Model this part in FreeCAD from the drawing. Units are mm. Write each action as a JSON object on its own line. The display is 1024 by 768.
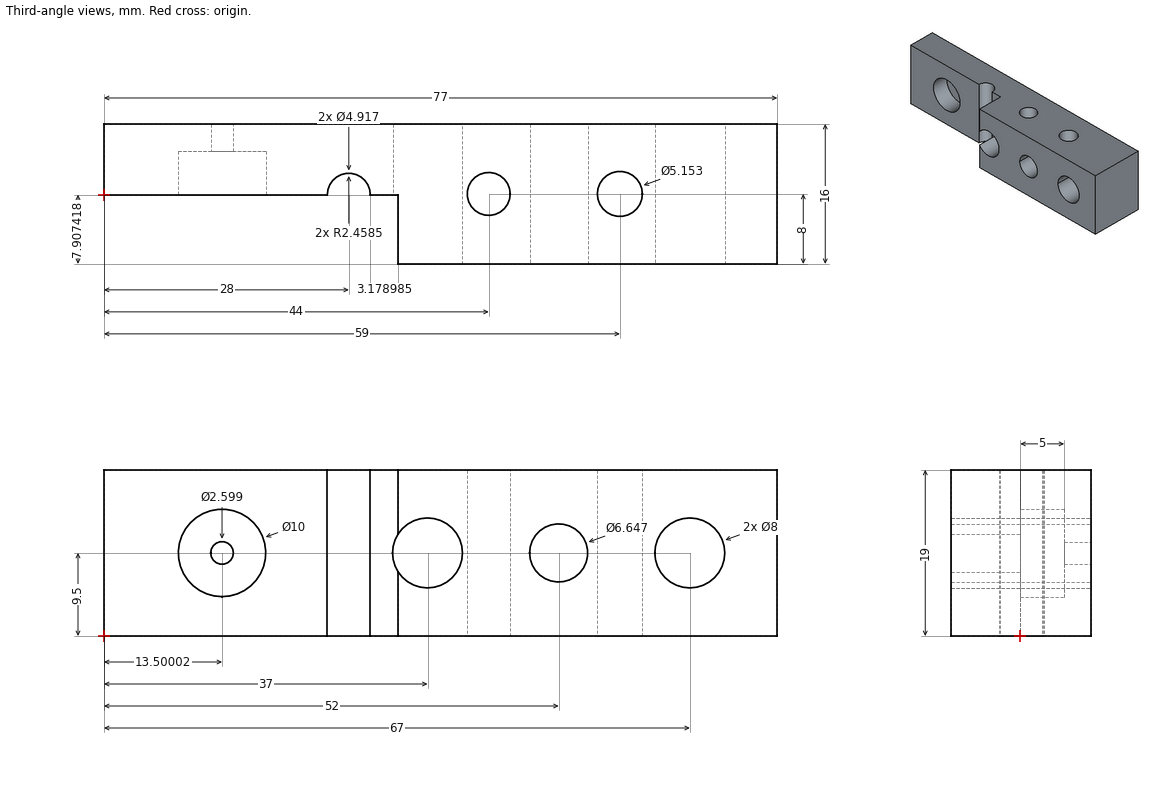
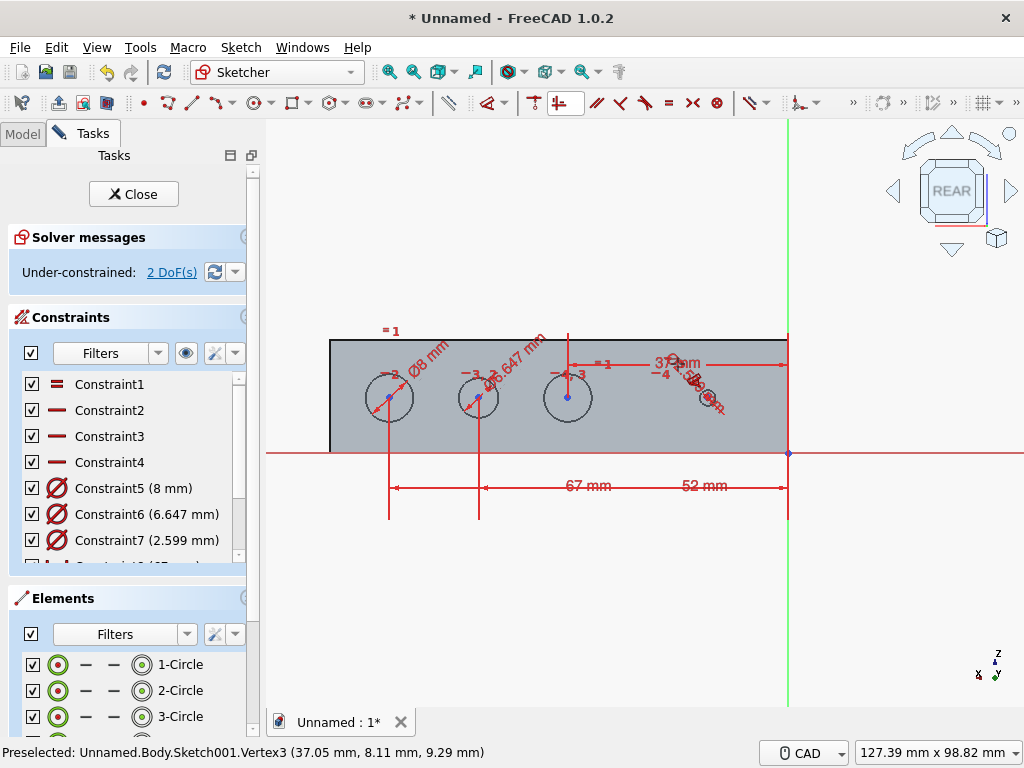
{"action": "left_click", "coordinate": [389, 398]}
{"action": "left_click", "coordinate": [822, 426]}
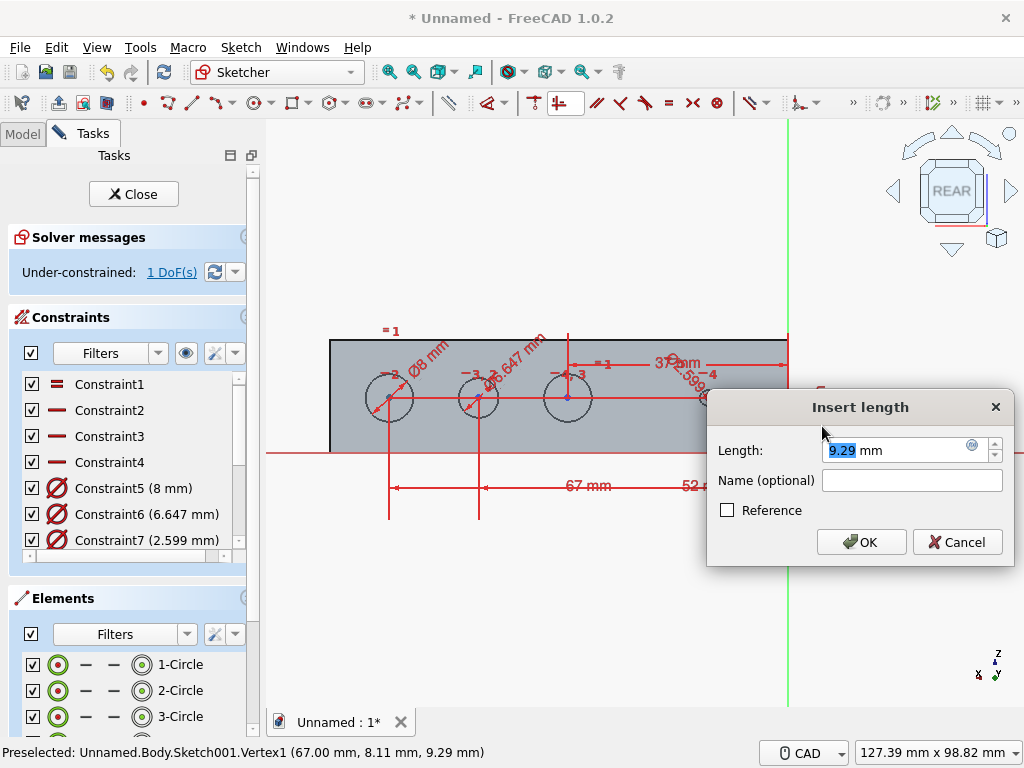
{"action": "type", "text": "9.5"}
{"action": "key", "text": "Return"}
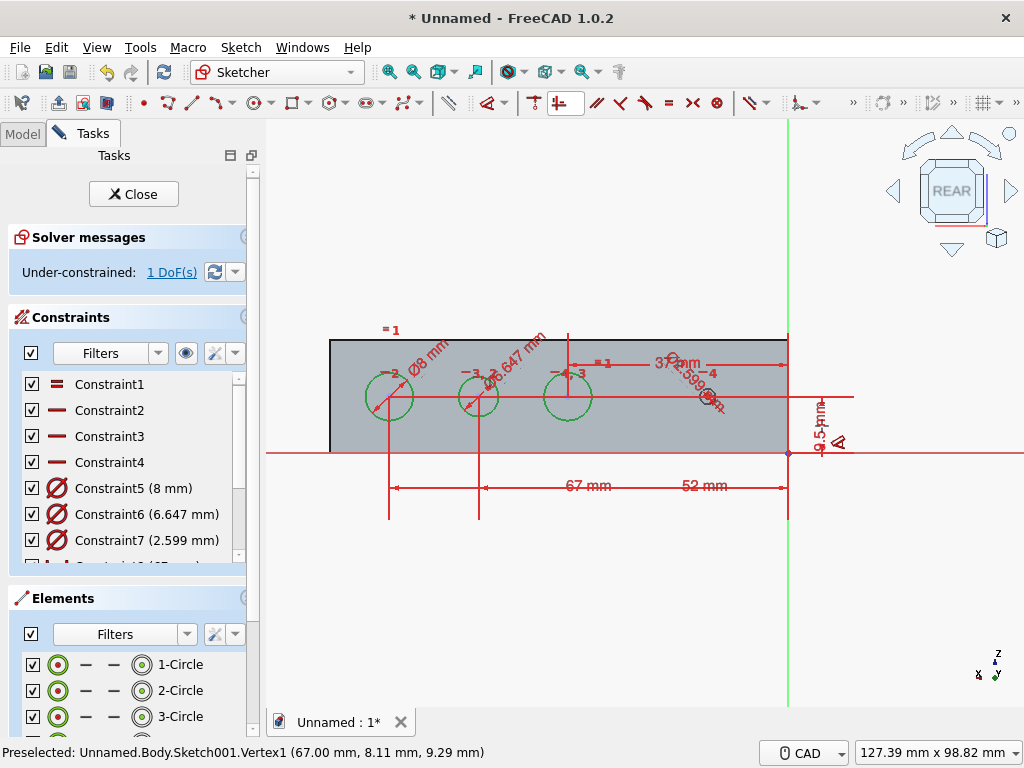
{"action": "left_click", "coordinate": [708, 397]}
{"action": "left_click", "coordinate": [748, 363]}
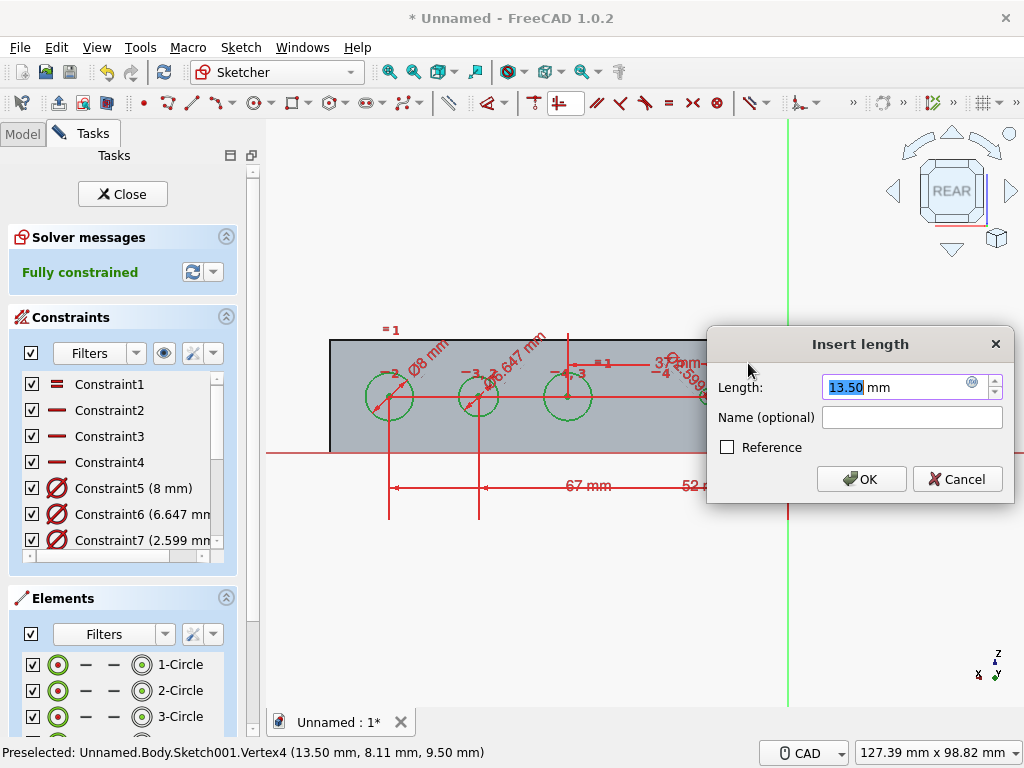
{"action": "type", "text": "13.50002"}
{"action": "key", "text": "Return"}
{"action": "key", "text": "Escape"}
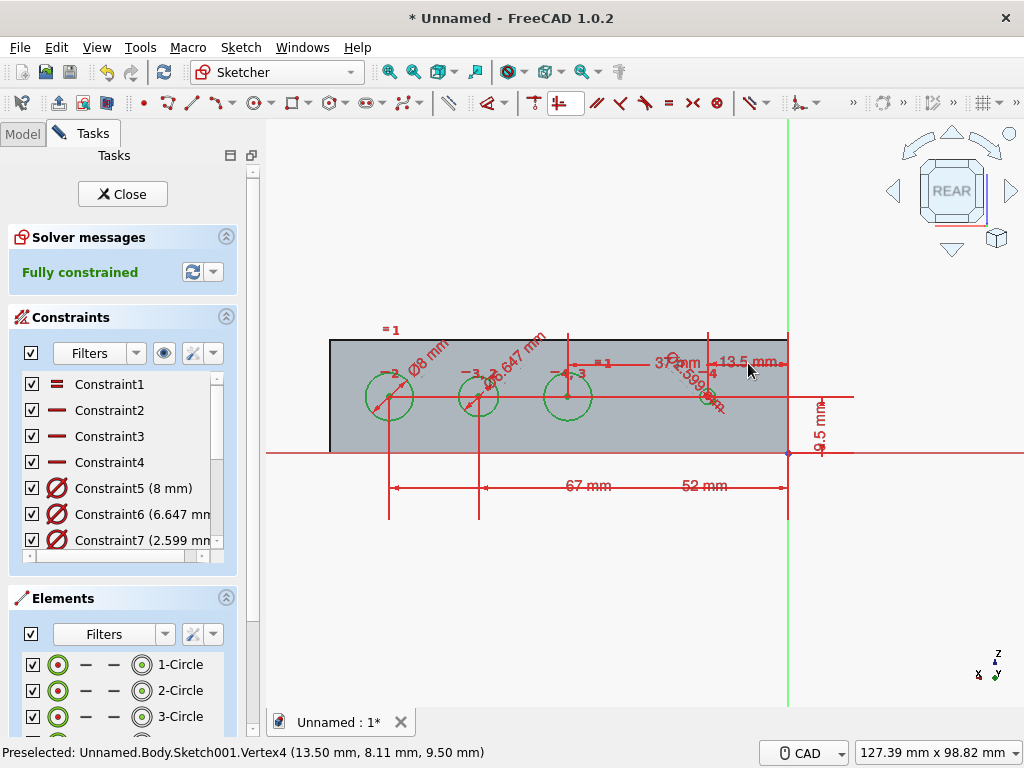
{"action": "left_click", "coordinate": [123, 194]}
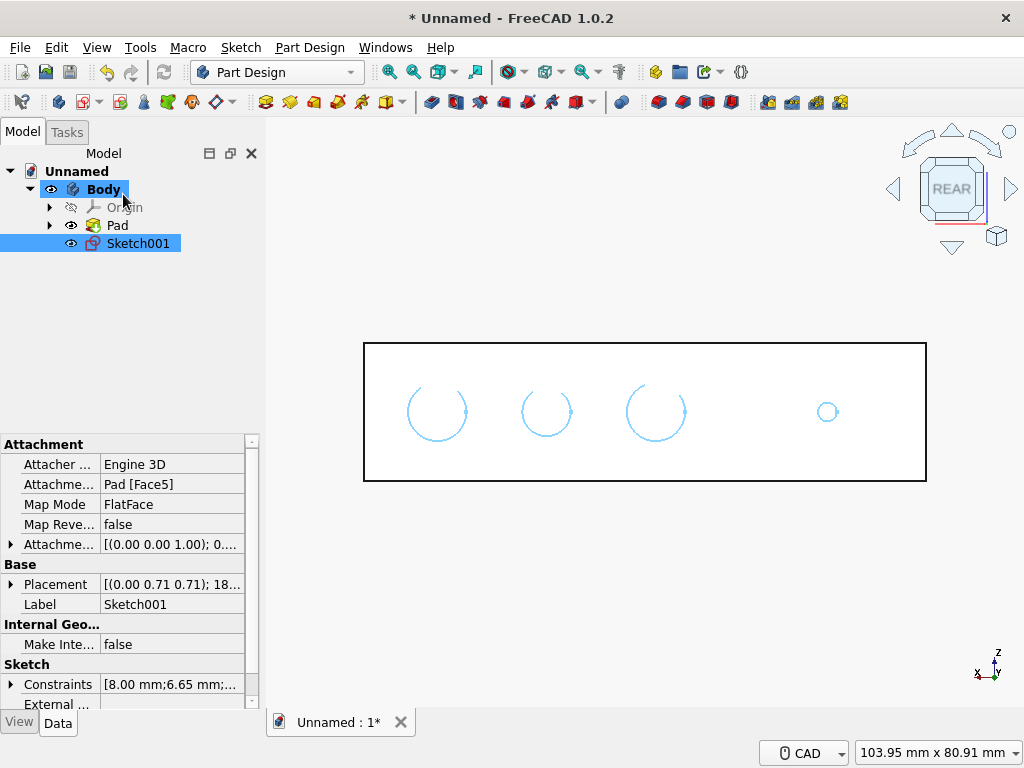
{"action": "left_click", "coordinate": [432, 102]}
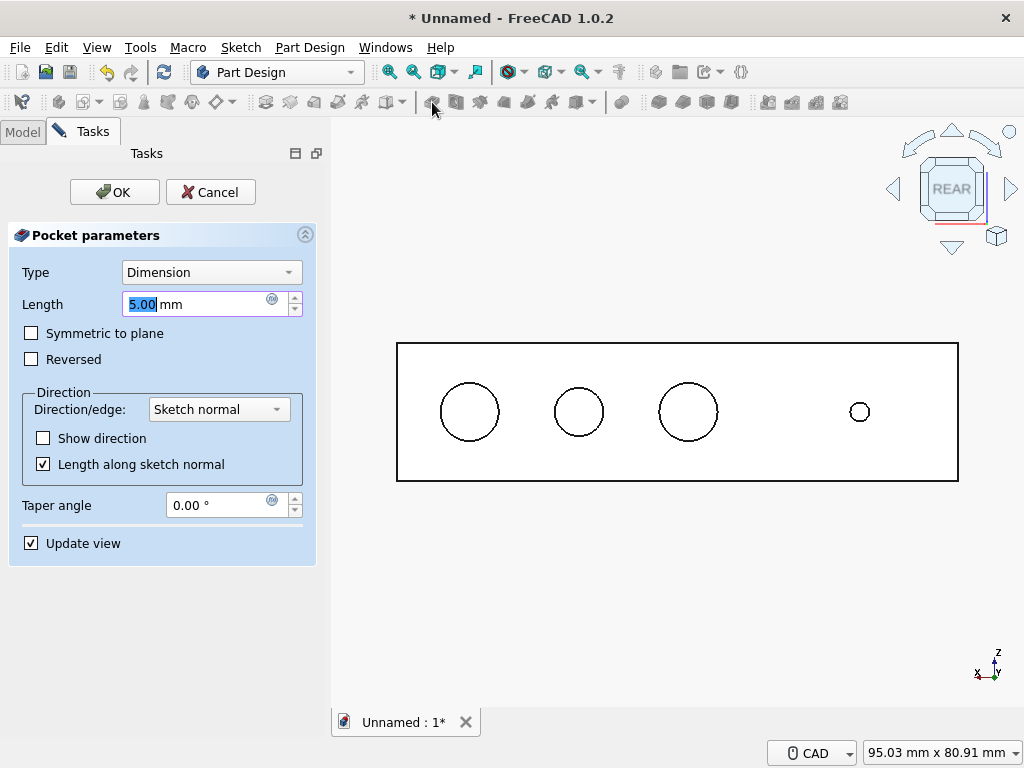
{"action": "left_click", "coordinate": [212, 272]}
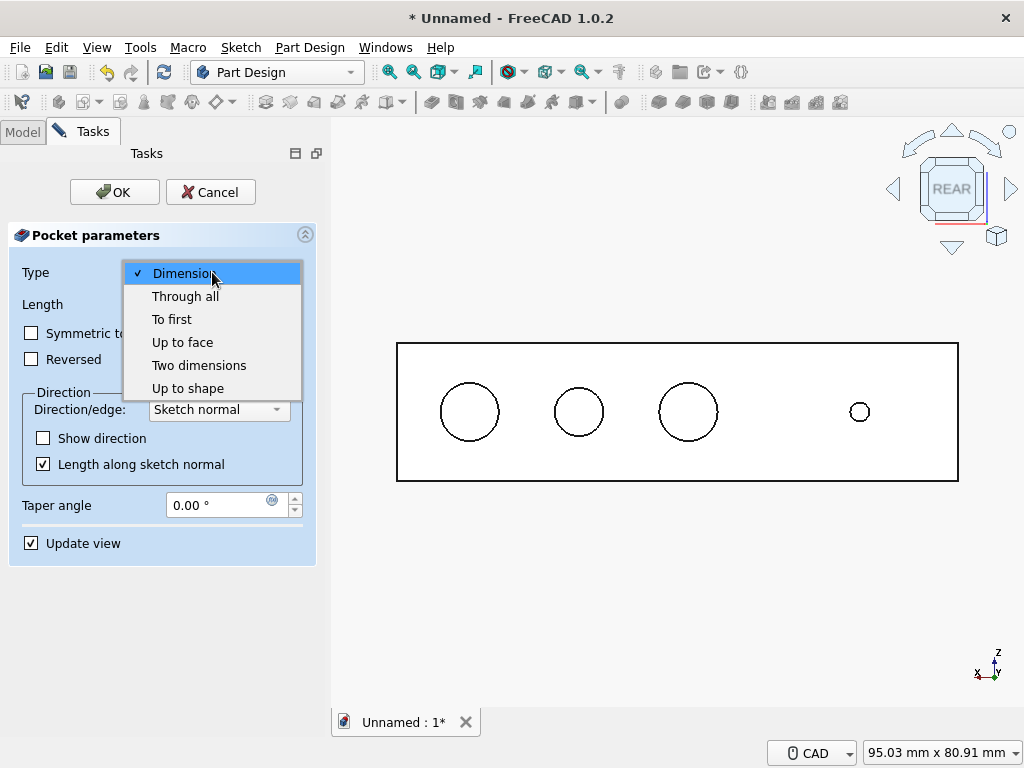
{"action": "left_click", "coordinate": [212, 296]}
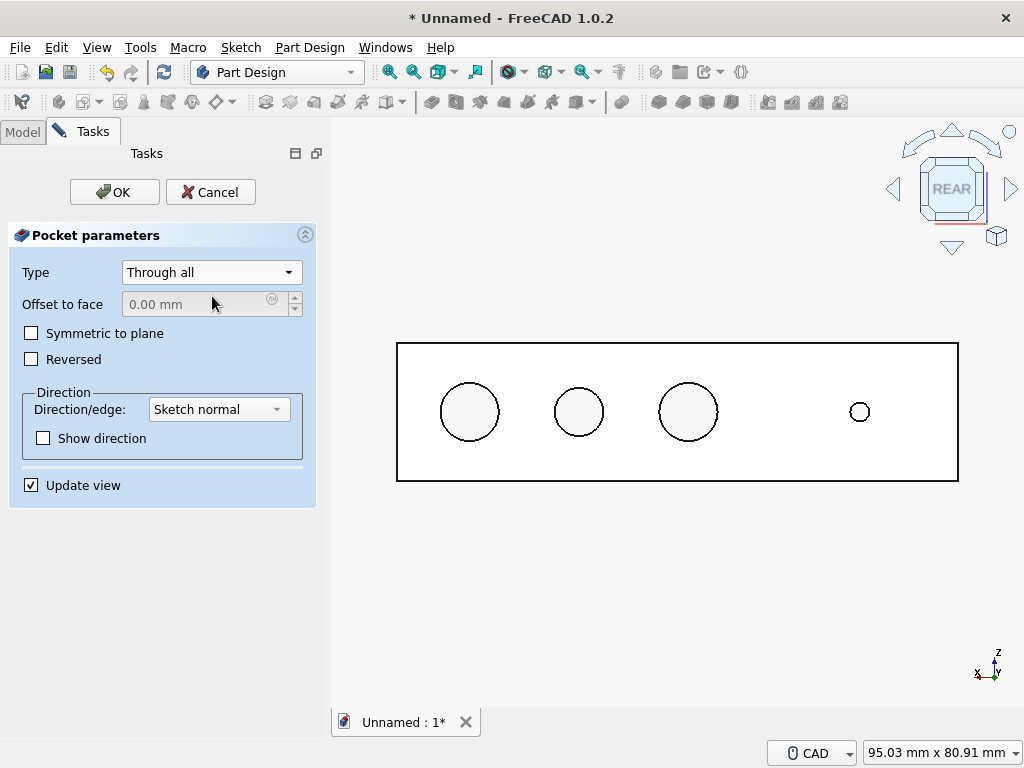
{"action": "left_click", "coordinate": [115, 192]}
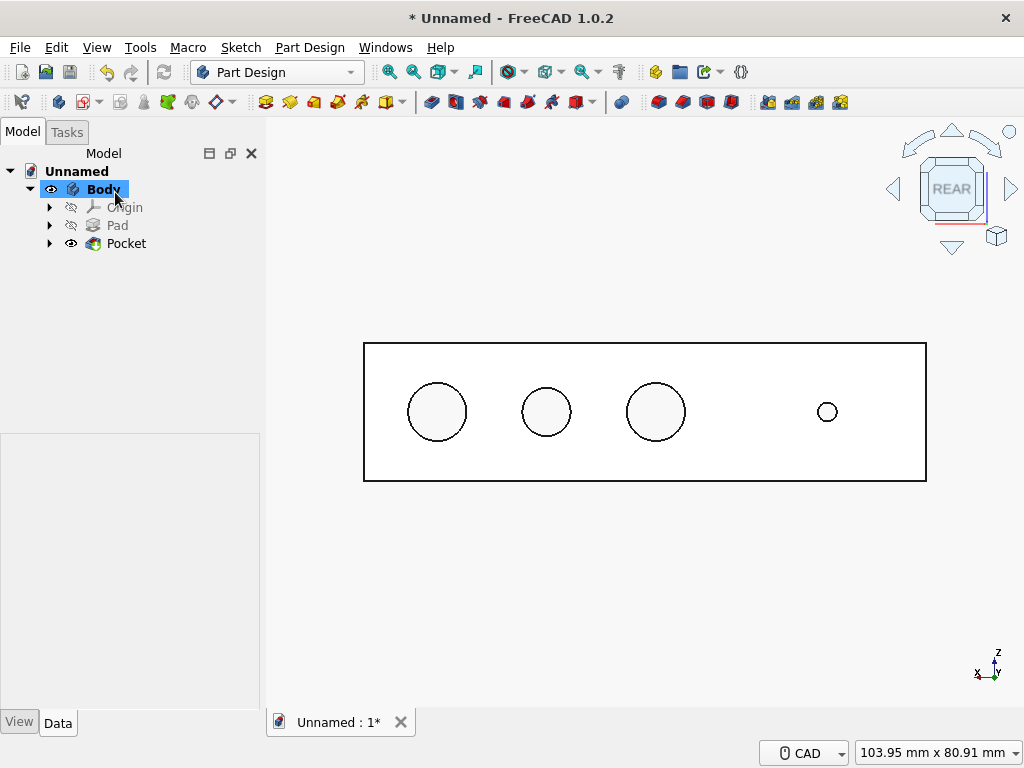
{"action": "key", "text": "0"}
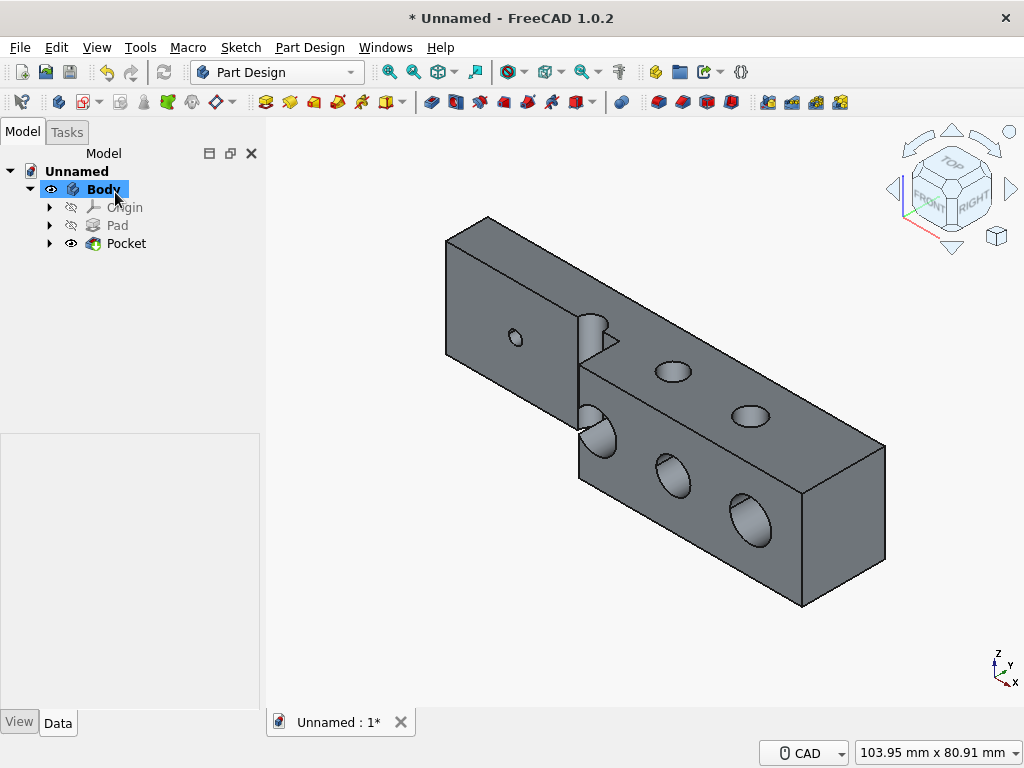
{"action": "left_click", "coordinate": [474, 297]}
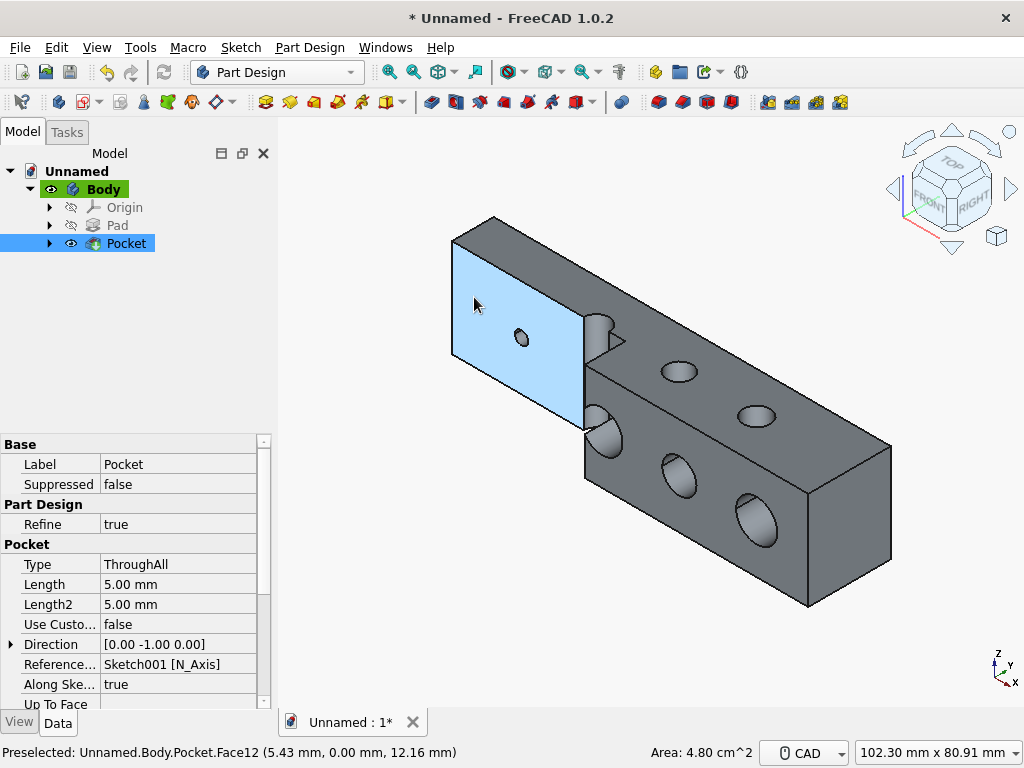
{"action": "left_click", "coordinate": [84, 102]}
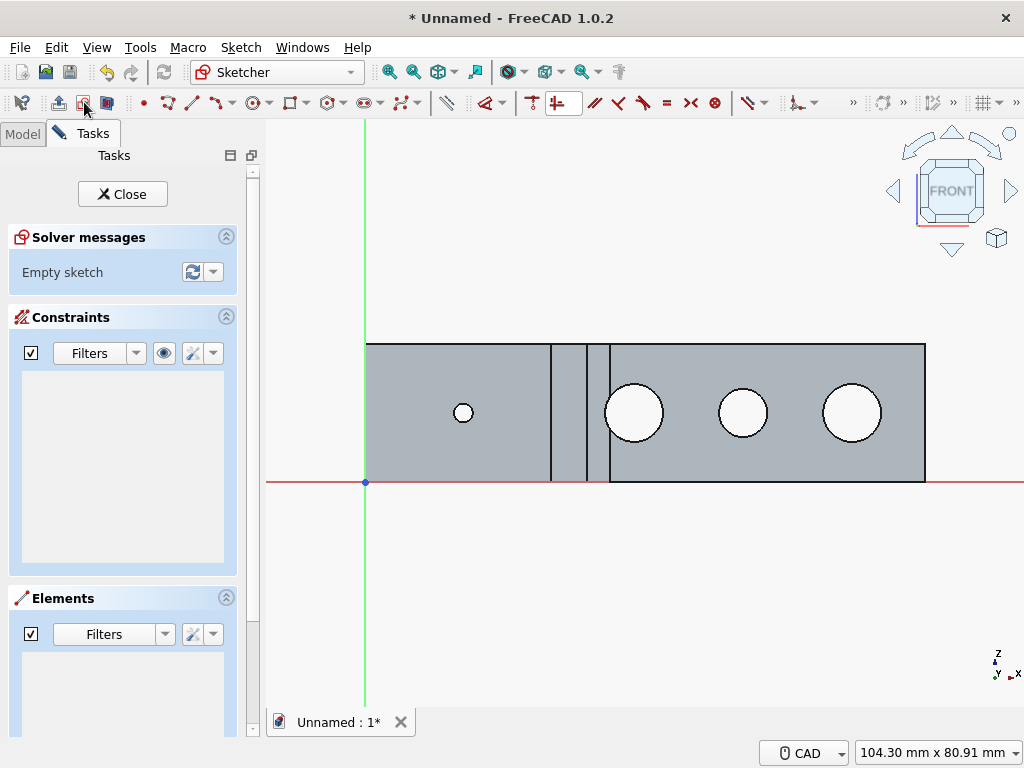
{"action": "scroll", "coordinate": [349, 439], "scroll_direction": "up", "scroll_amount": 5}